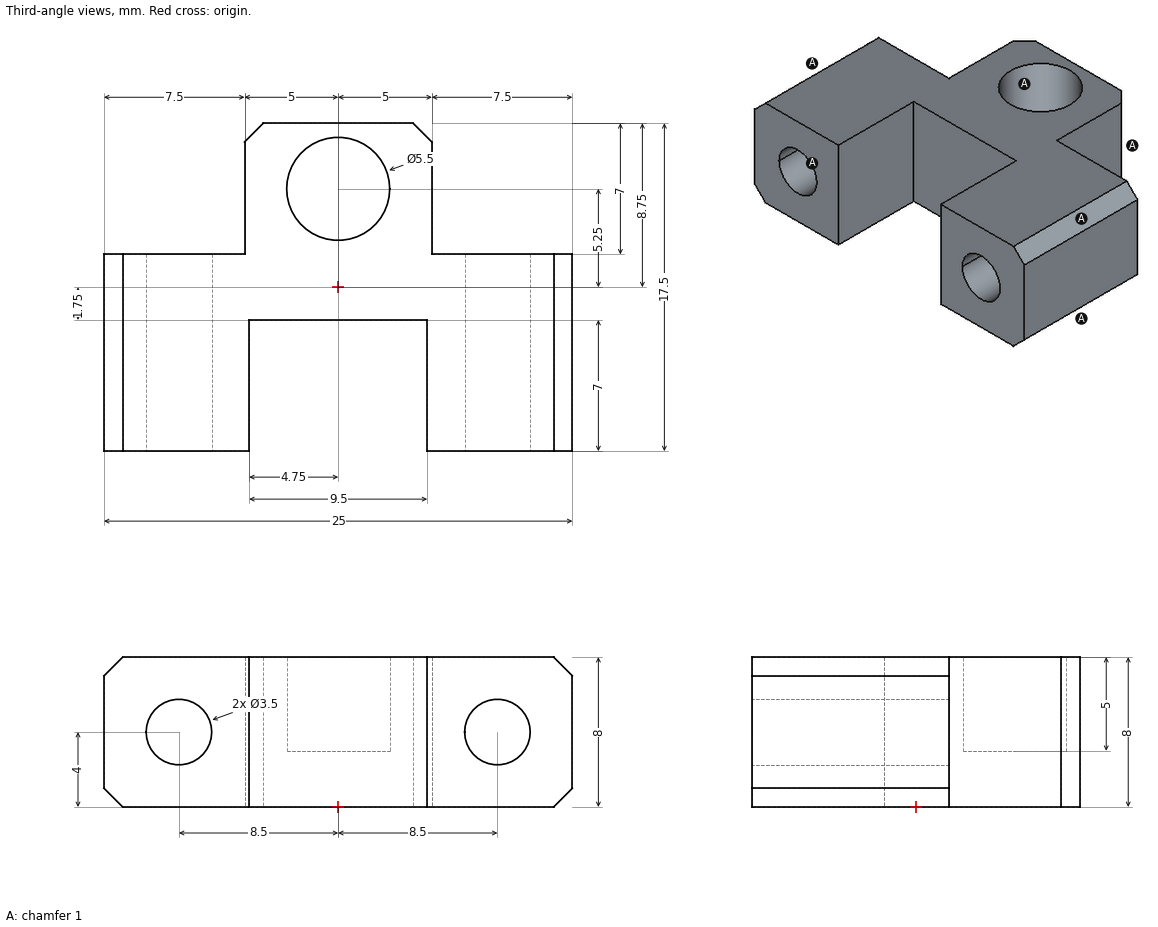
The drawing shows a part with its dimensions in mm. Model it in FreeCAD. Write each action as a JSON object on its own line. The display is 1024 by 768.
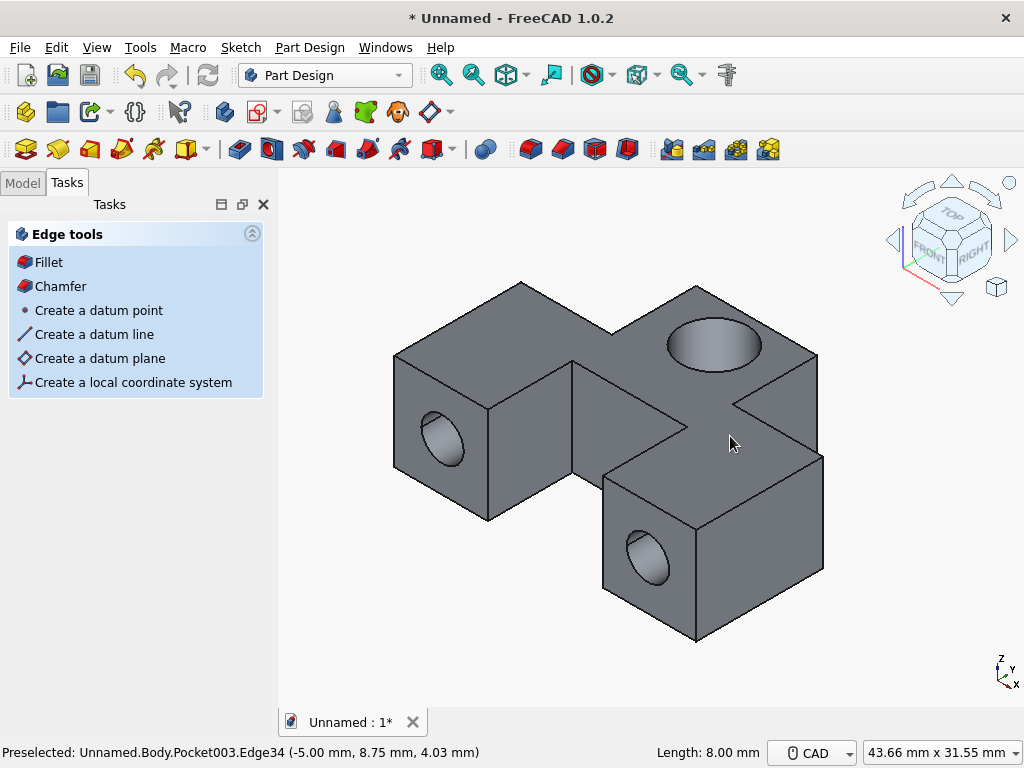
{"action": "left_click", "coordinate": [760, 492], "text": "ctrl"}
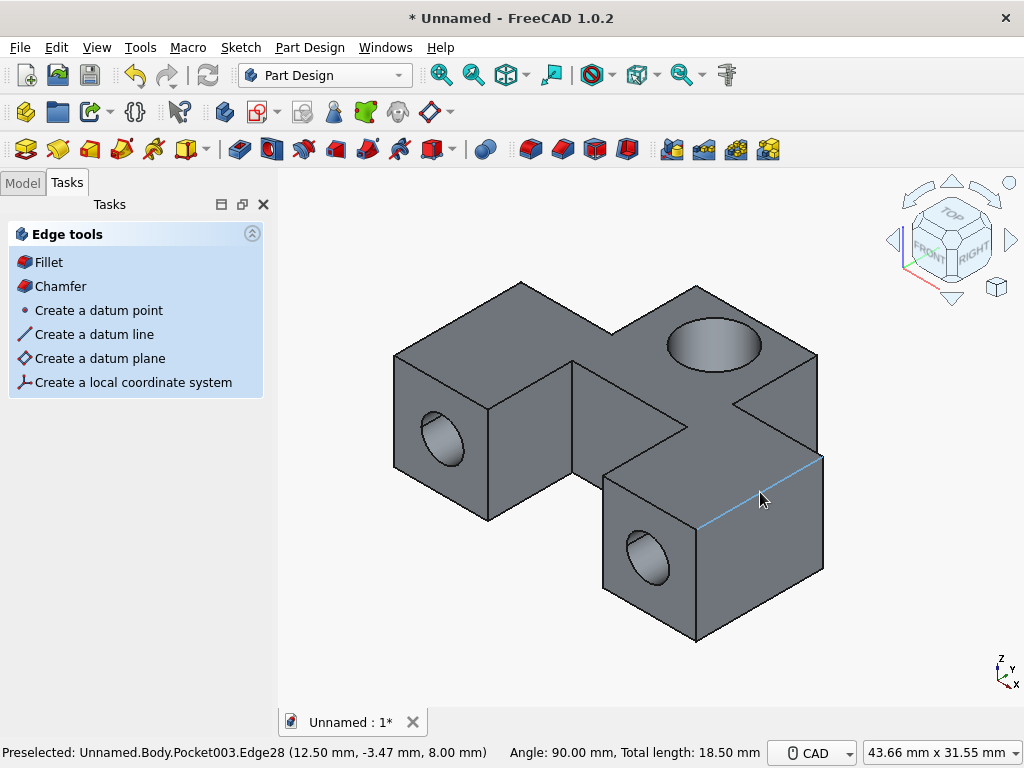
{"action": "key", "text": "2"}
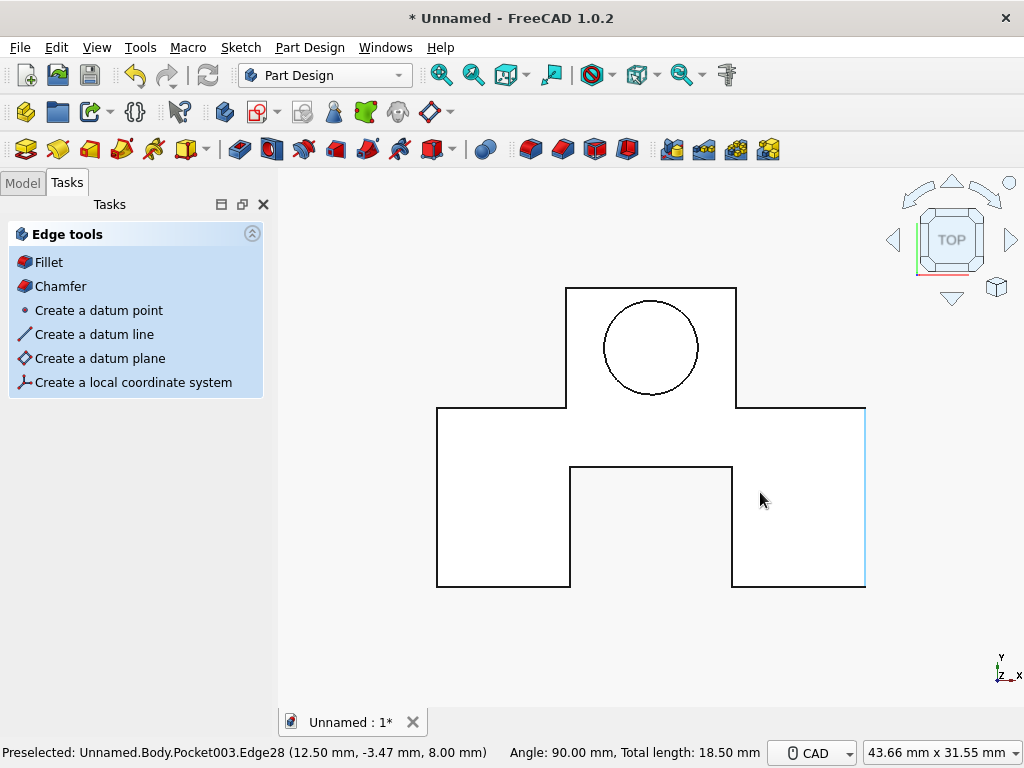
{"action": "left_click", "coordinate": [437, 496], "text": "ctrl"}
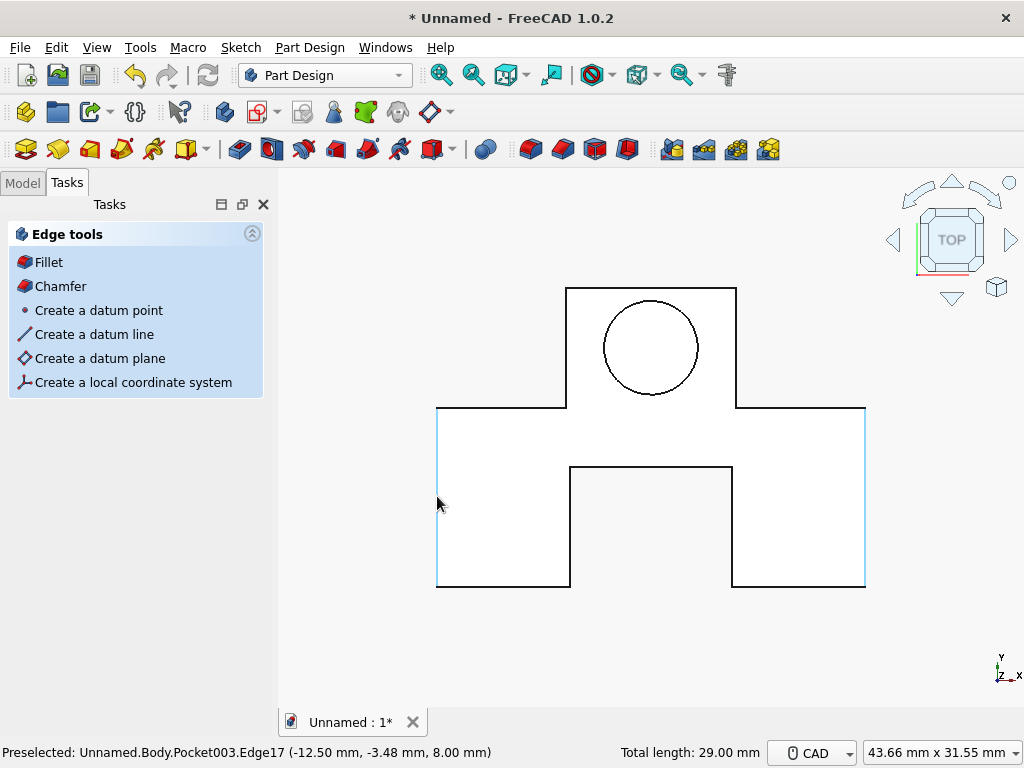
{"action": "key", "text": "1"}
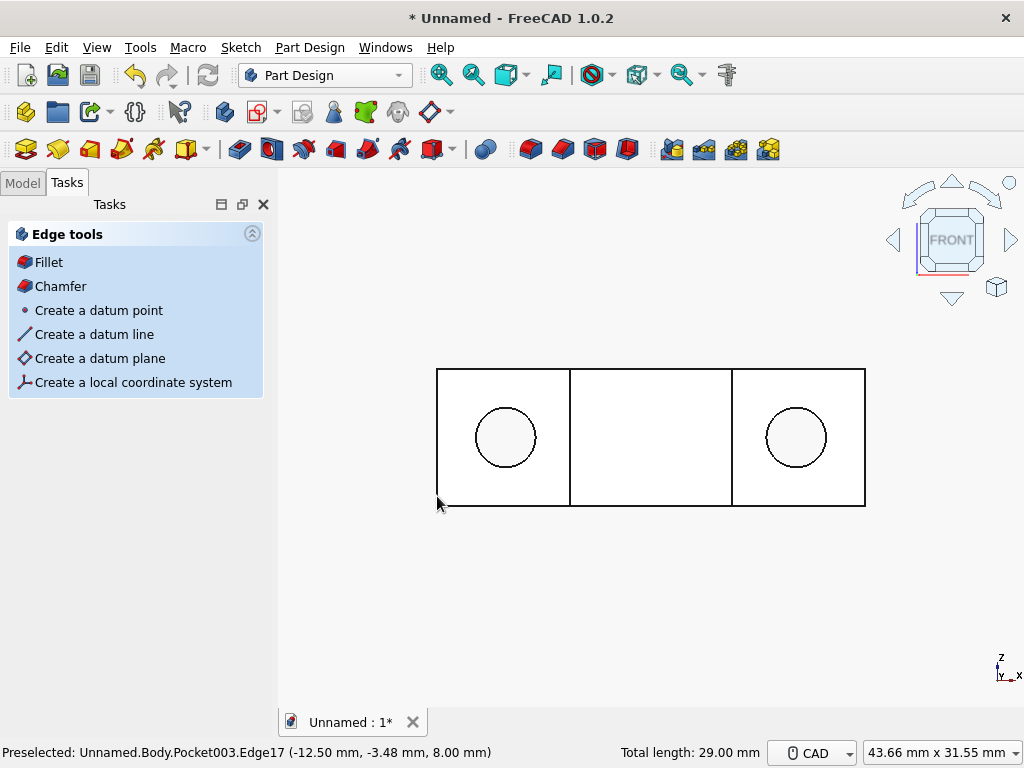
{"action": "key", "text": "3"}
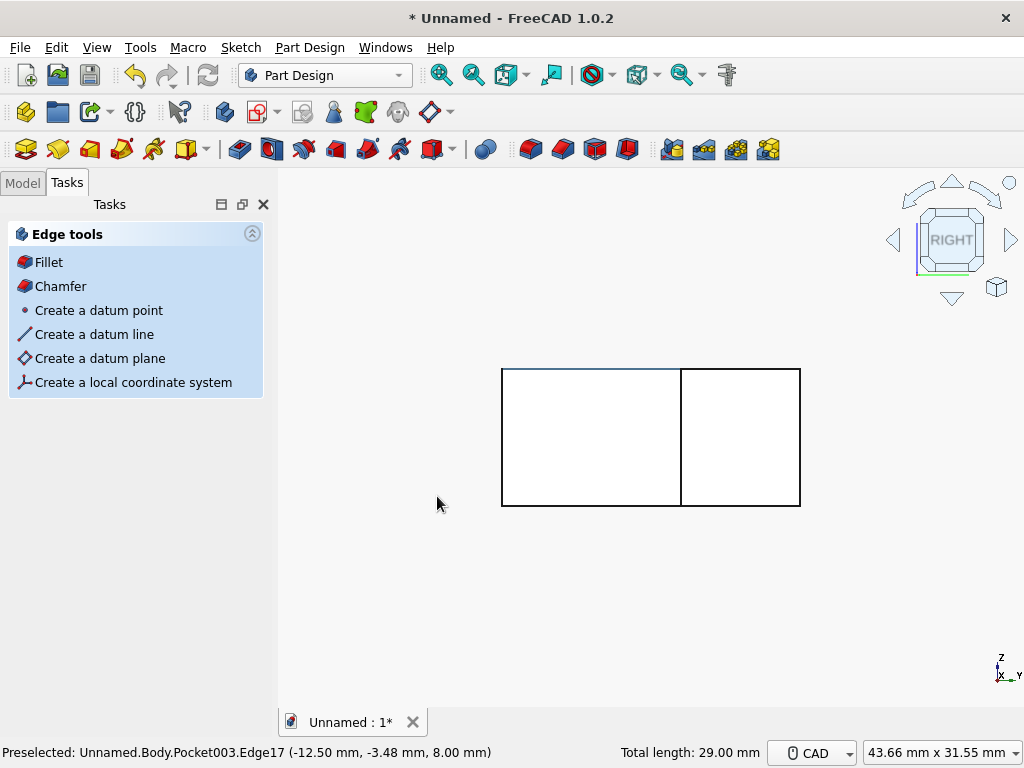
{"action": "left_click", "coordinate": [442, 76]}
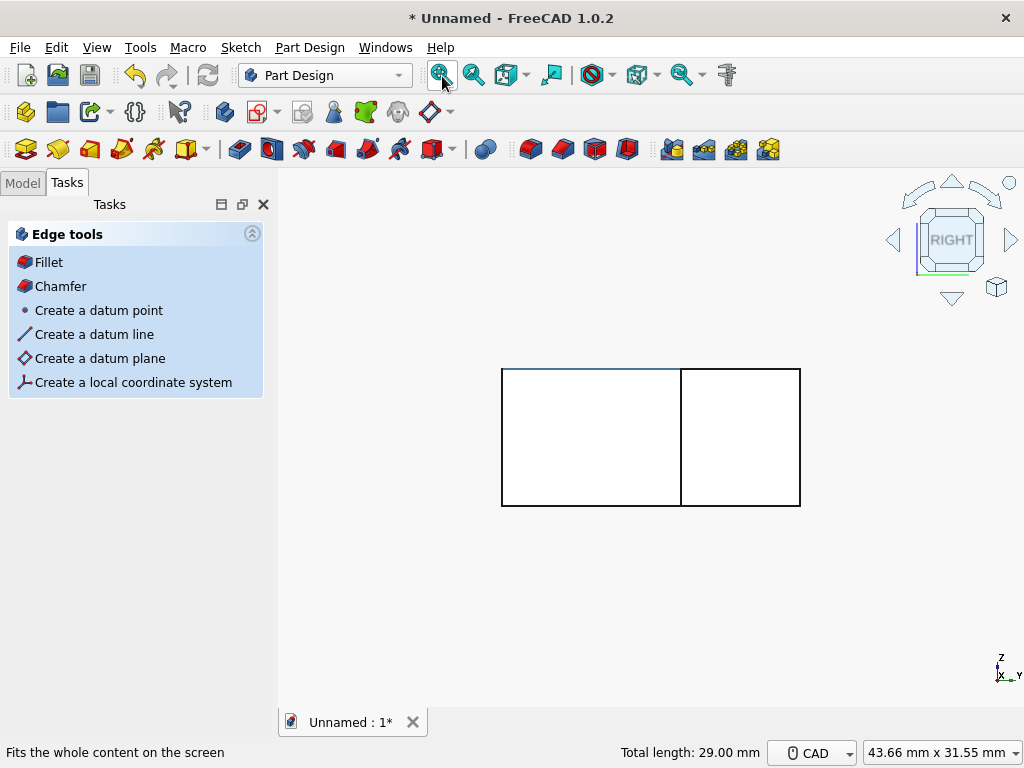
{"action": "left_click", "coordinate": [800, 436], "text": "ctrl"}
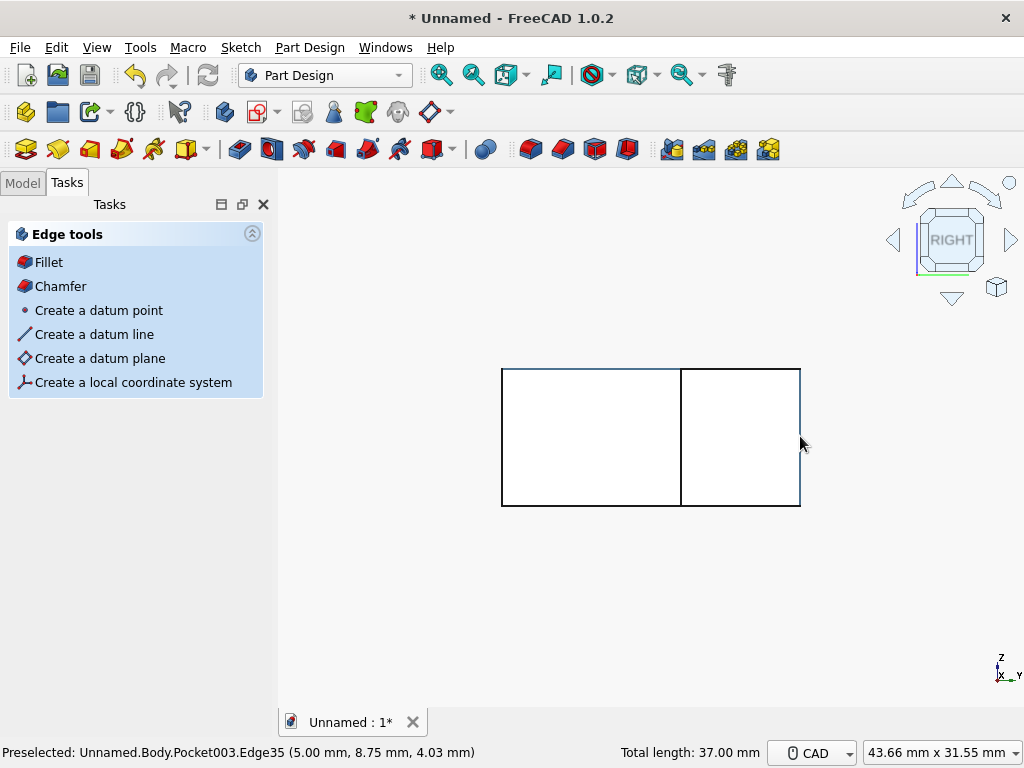
{"action": "left_click", "coordinate": [591, 505], "text": "ctrl"}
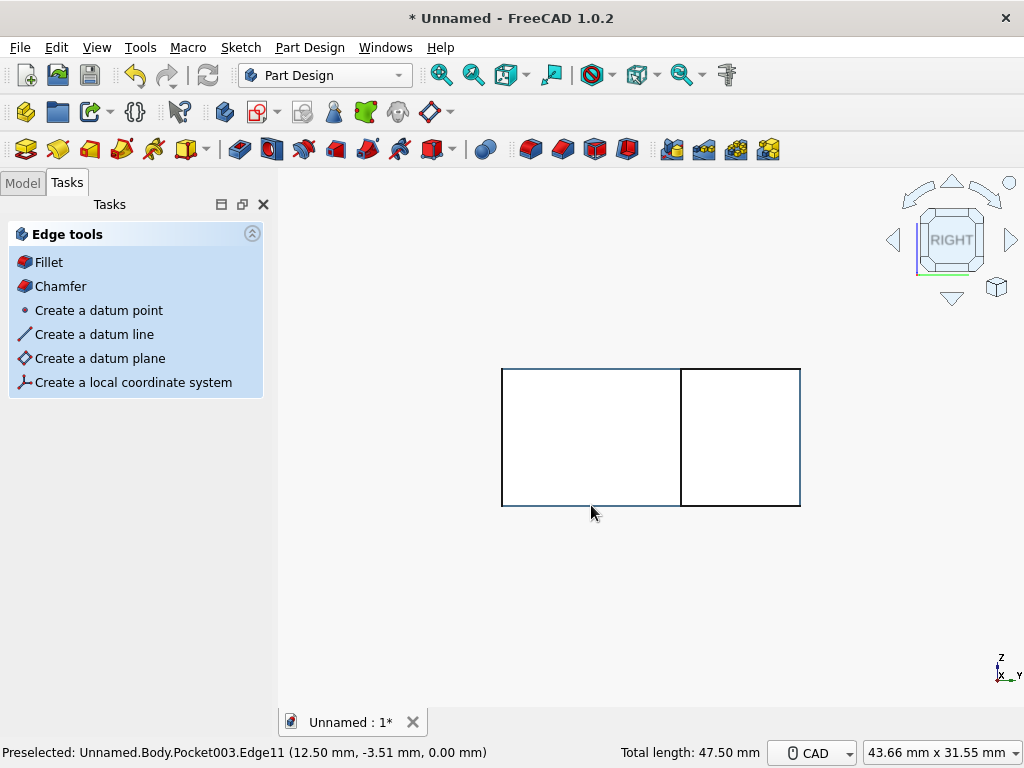
{"action": "key", "text": "5"}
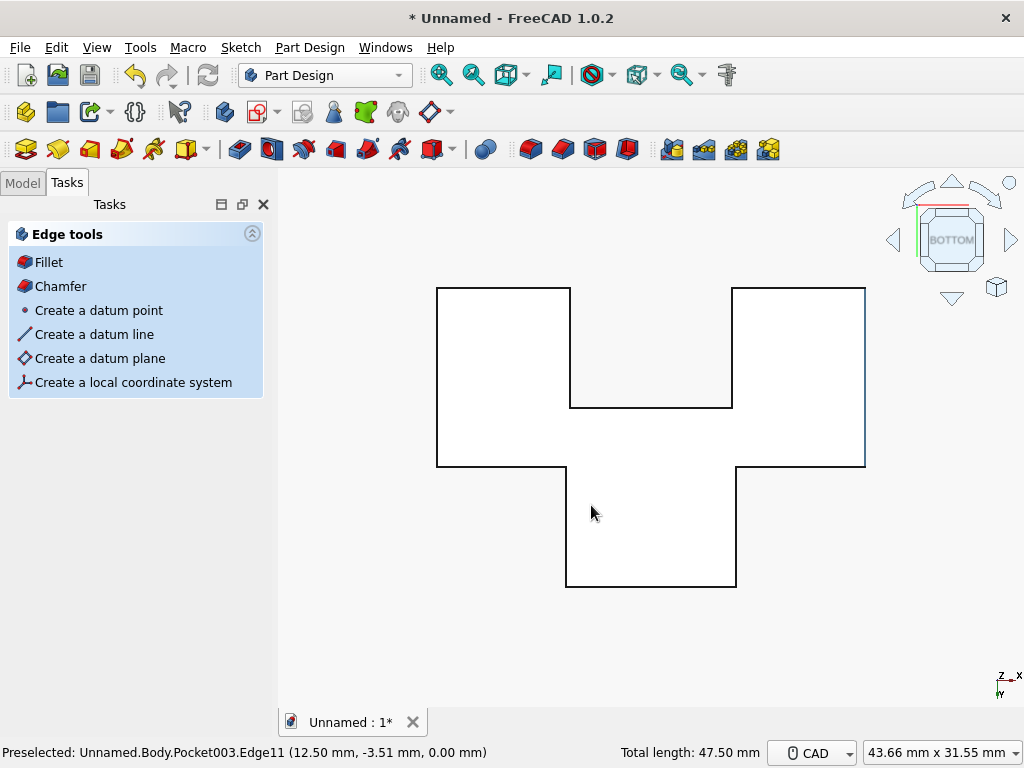
{"action": "left_click", "coordinate": [437, 377], "text": "ctrl"}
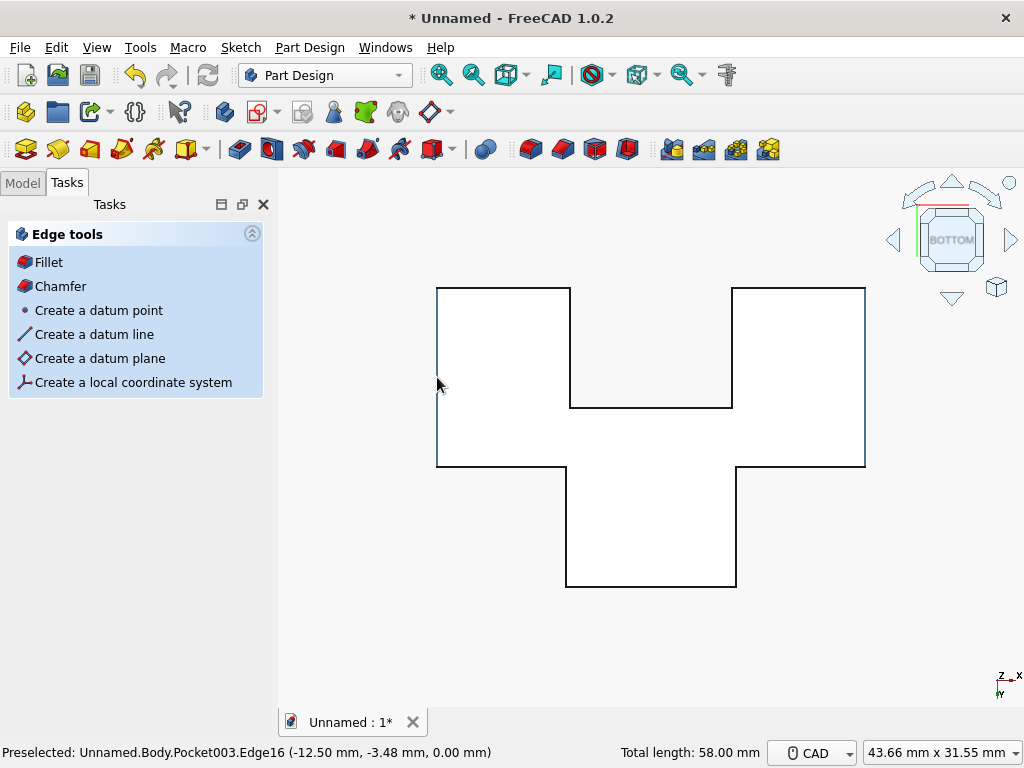
{"action": "left_click", "coordinate": [564, 150]}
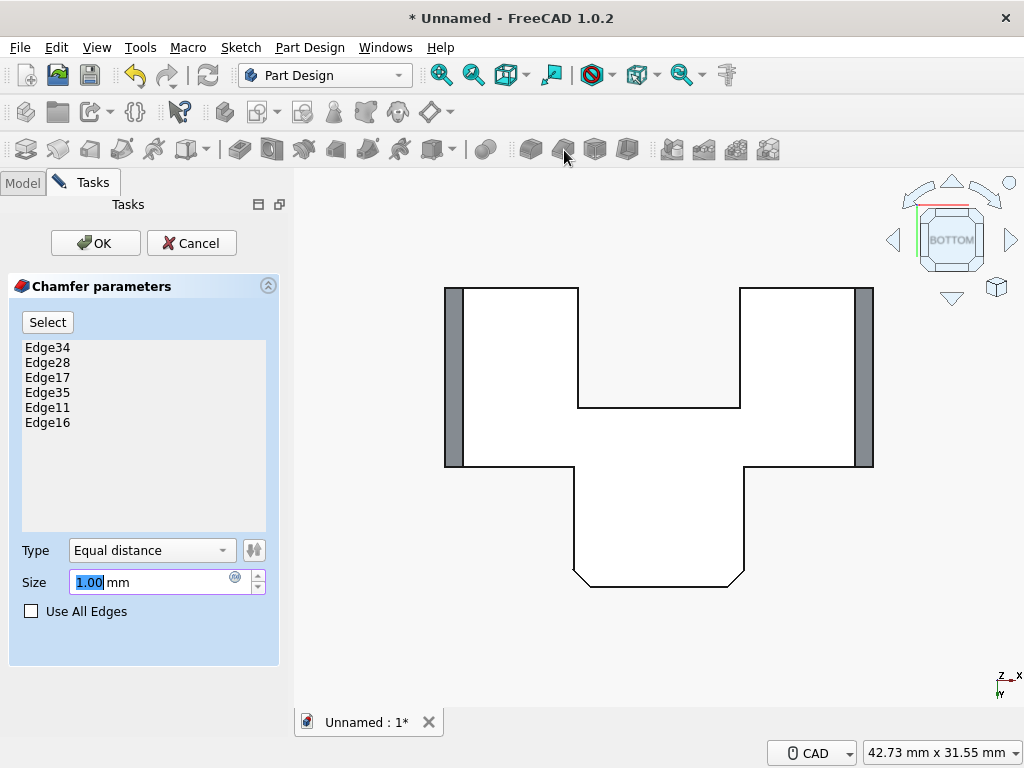
{"action": "type", "text": "1"}
{"action": "key", "text": "Tab"}